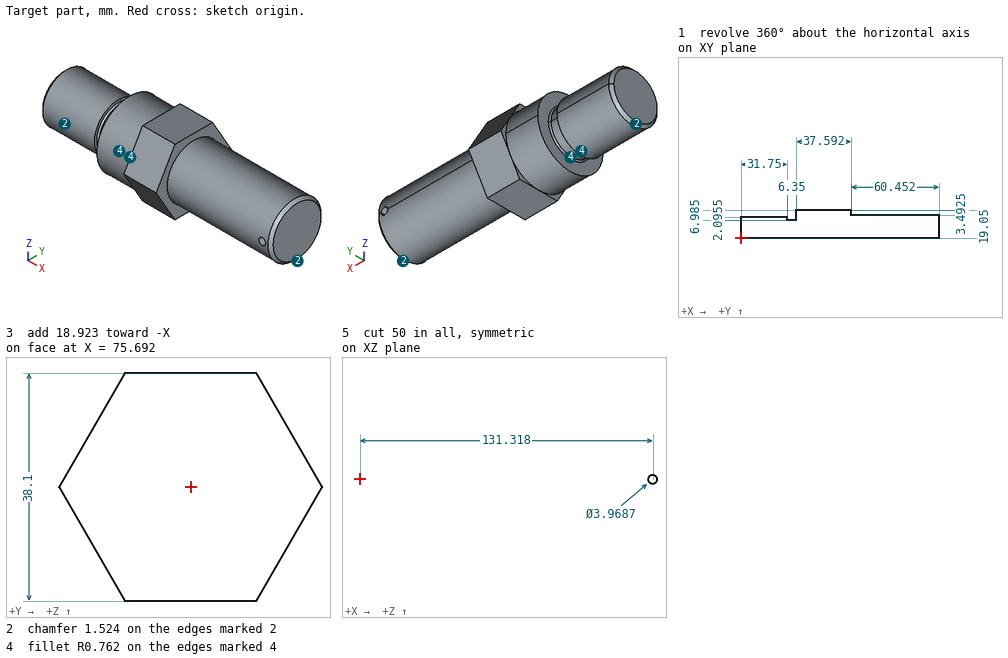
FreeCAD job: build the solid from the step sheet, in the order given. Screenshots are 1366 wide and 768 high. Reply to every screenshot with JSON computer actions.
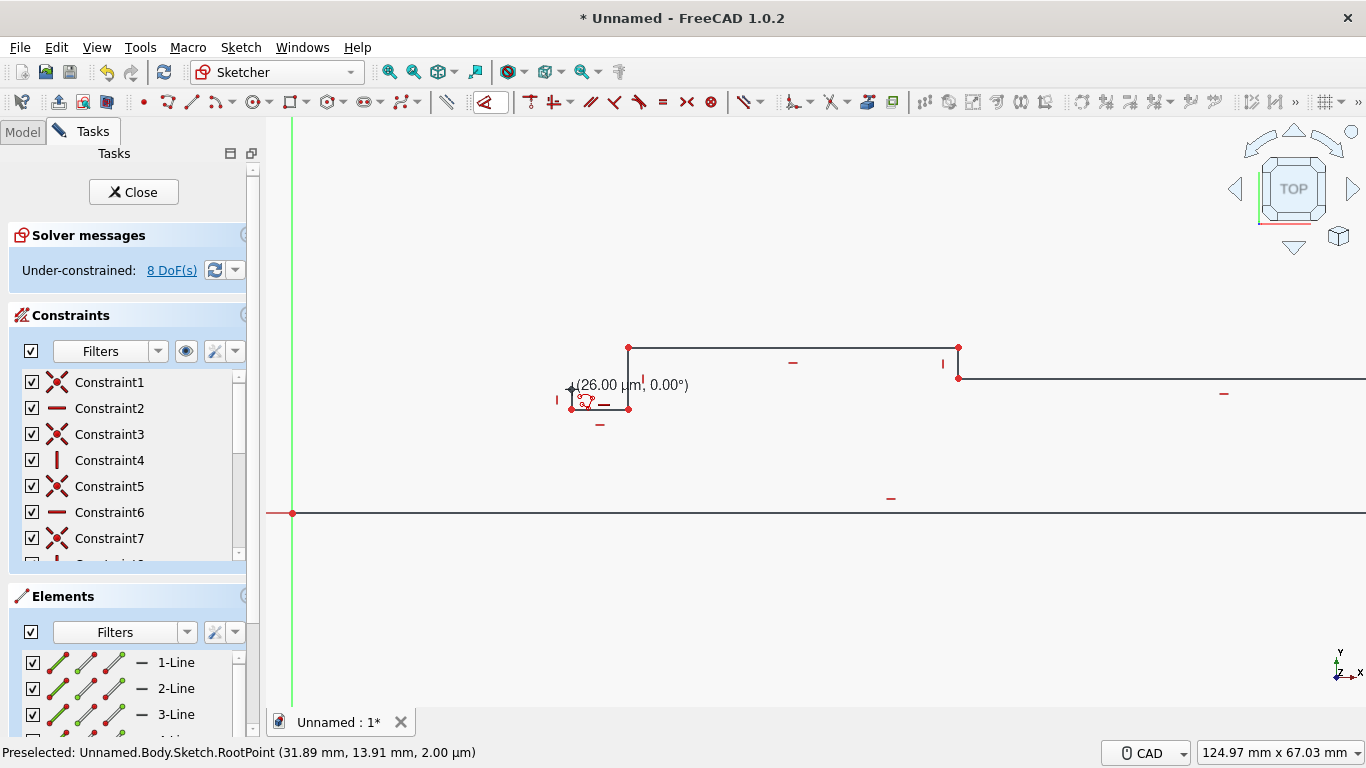
{"action": "scroll", "coordinate": [572, 391], "scroll_direction": "down", "scroll_amount": 3}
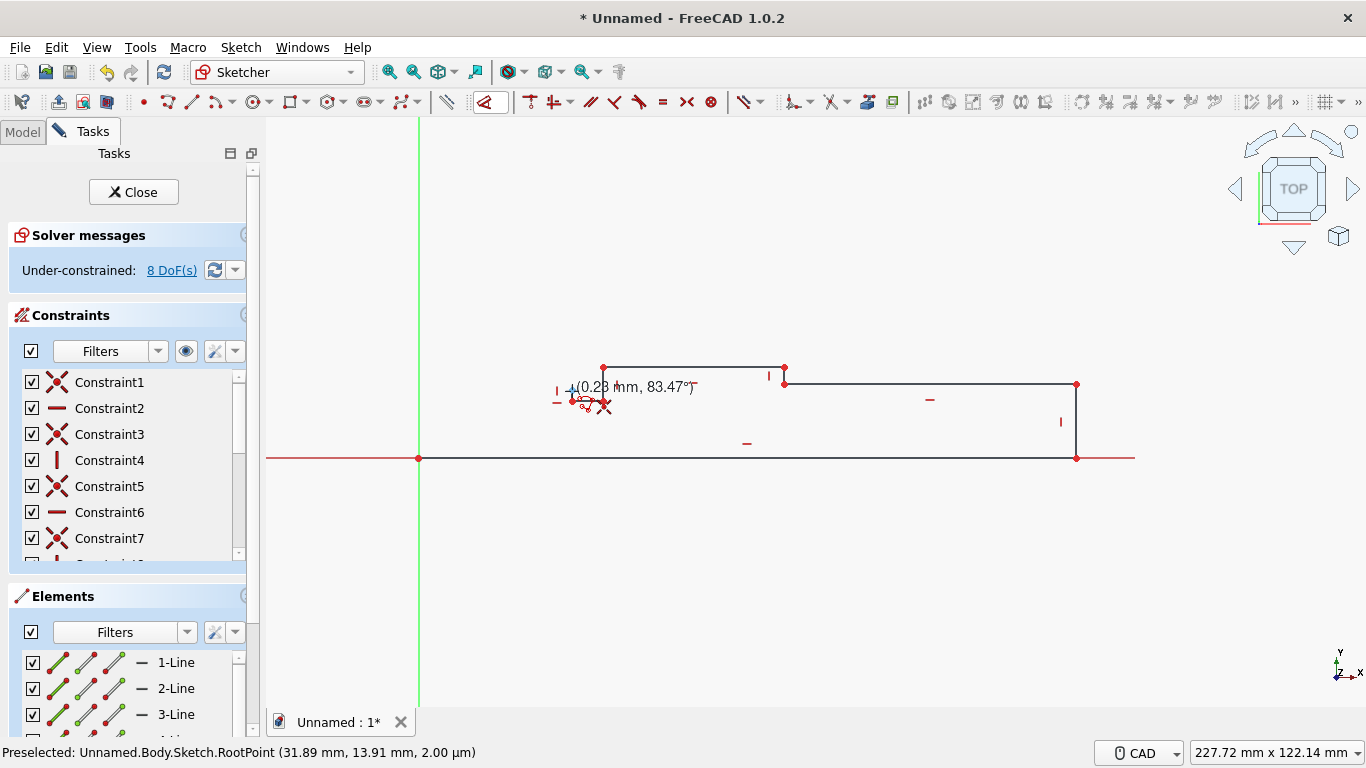
{"action": "left_click", "coordinate": [428, 390]}
{"action": "left_click", "coordinate": [419, 458]}
{"action": "key", "text": "Escape"}
{"action": "key", "text": "Escape"}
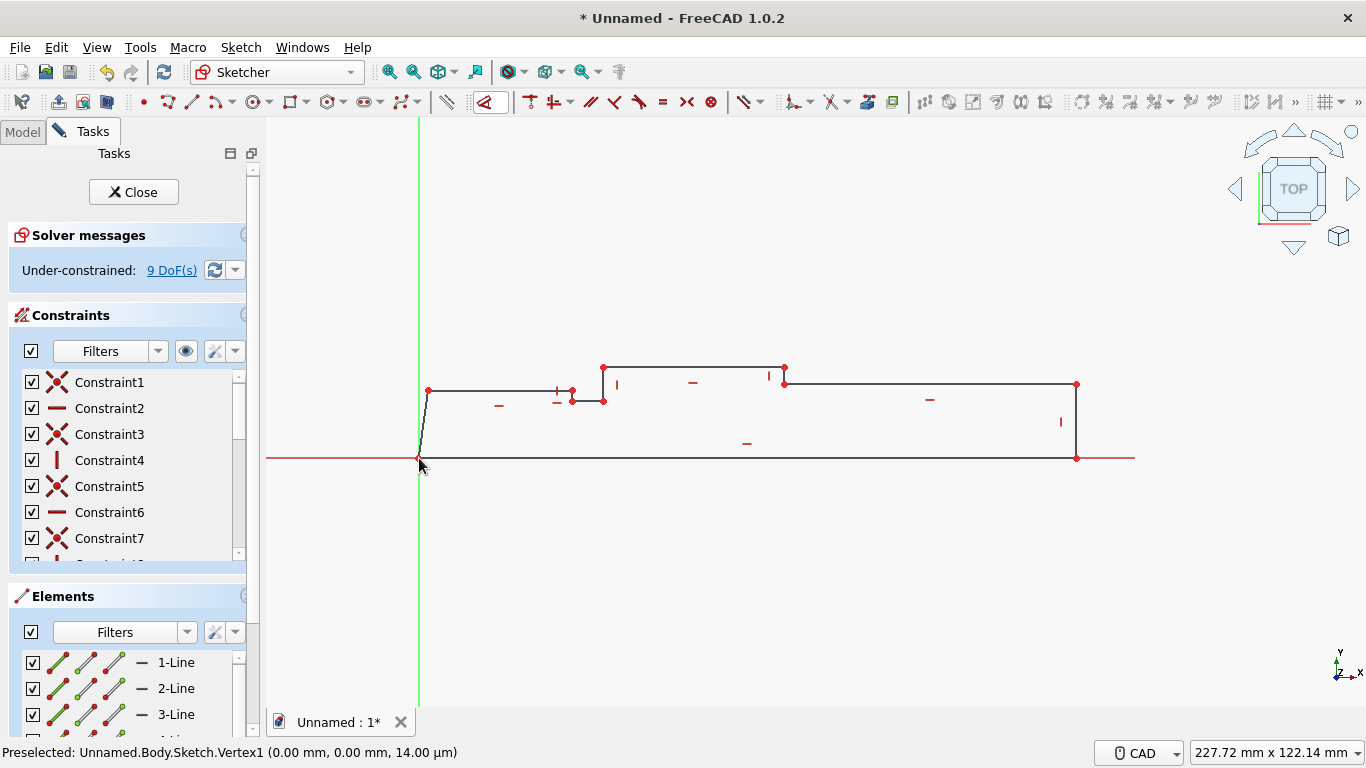
{"action": "left_click", "coordinate": [421, 438]}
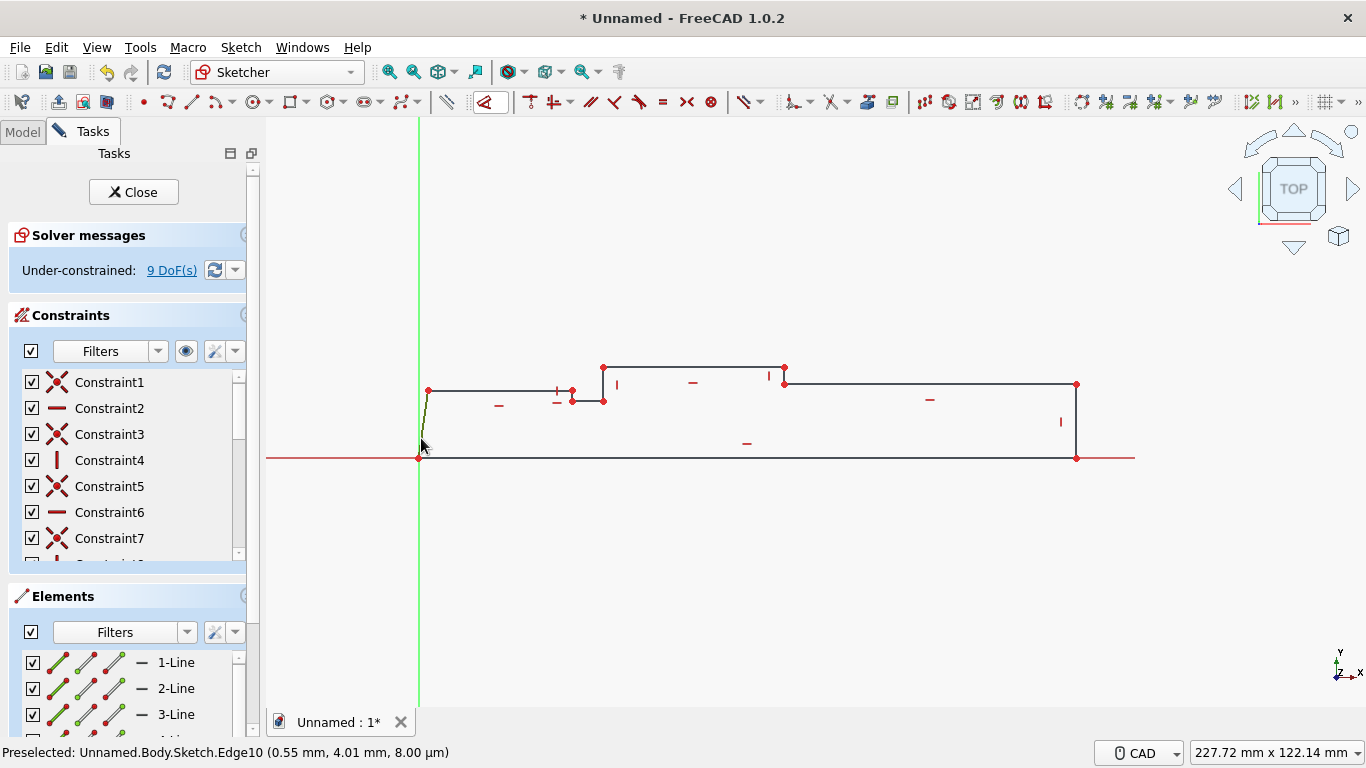
{"action": "key", "text": "v"}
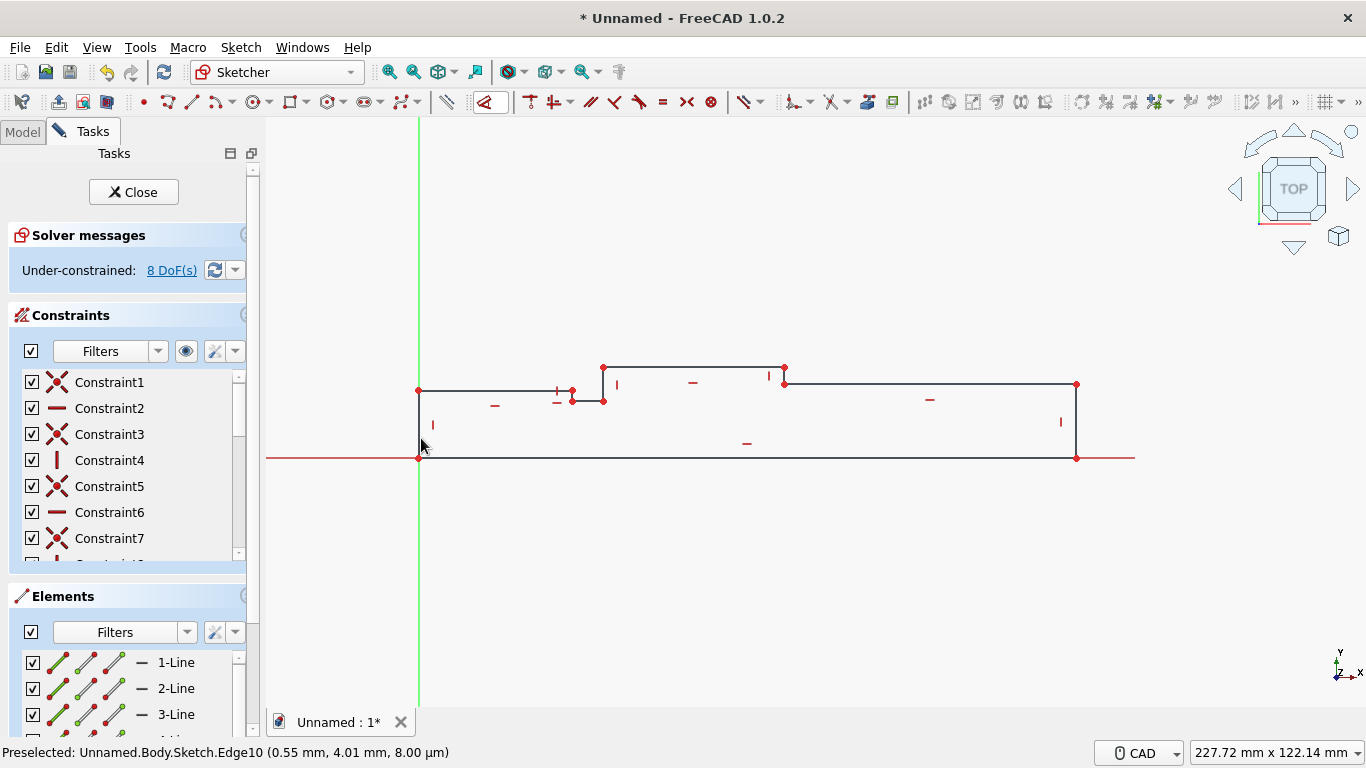
{"action": "key", "text": "d"}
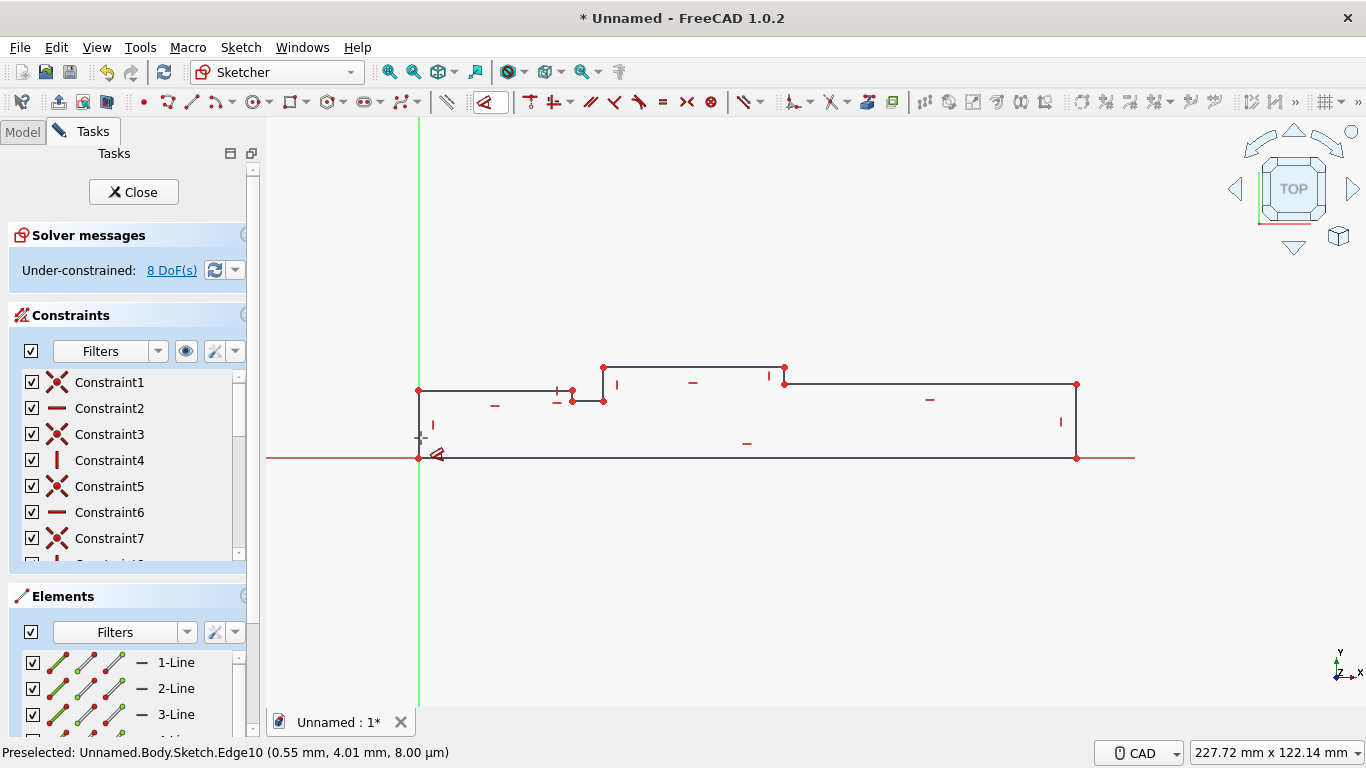
{"action": "scroll", "coordinate": [594, 401], "scroll_direction": "up", "scroll_amount": 2}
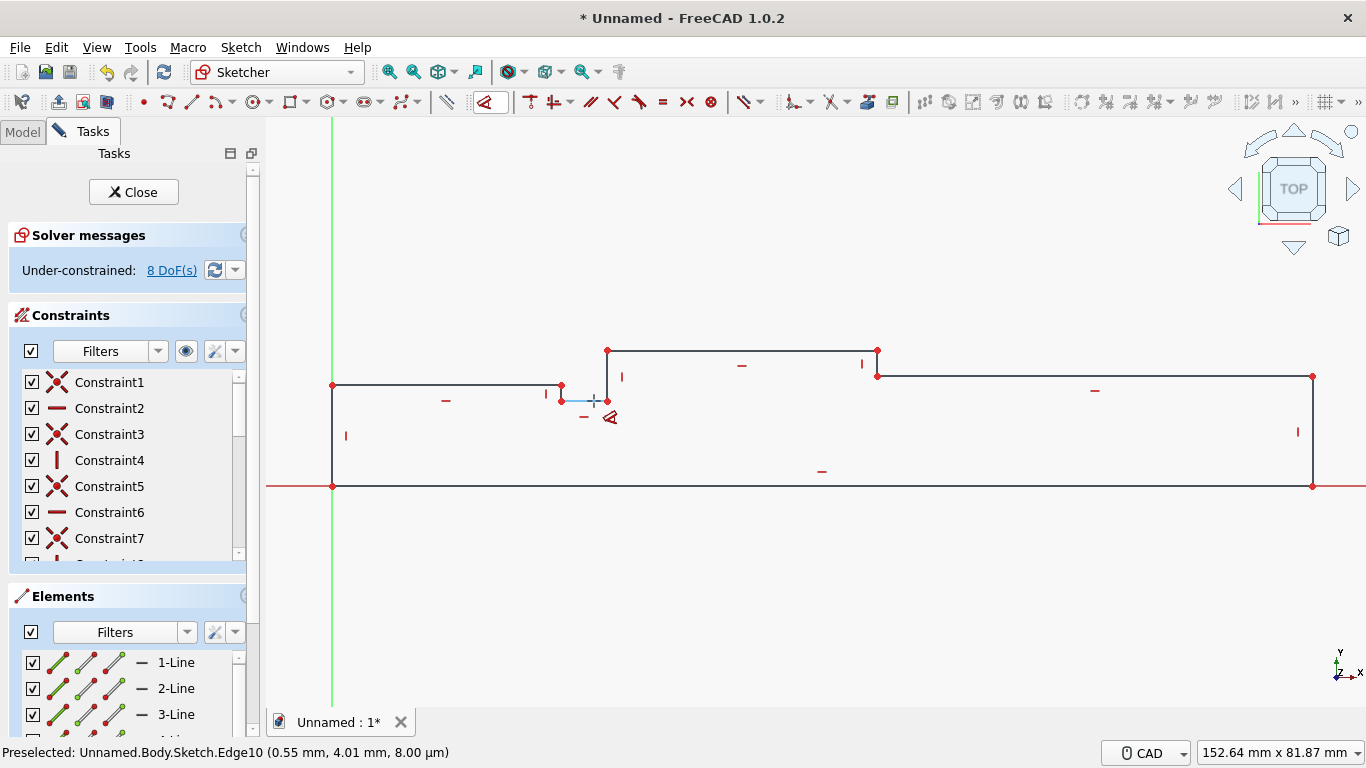
{"action": "left_click", "coordinate": [593, 401]}
{"action": "left_click", "coordinate": [584, 367]}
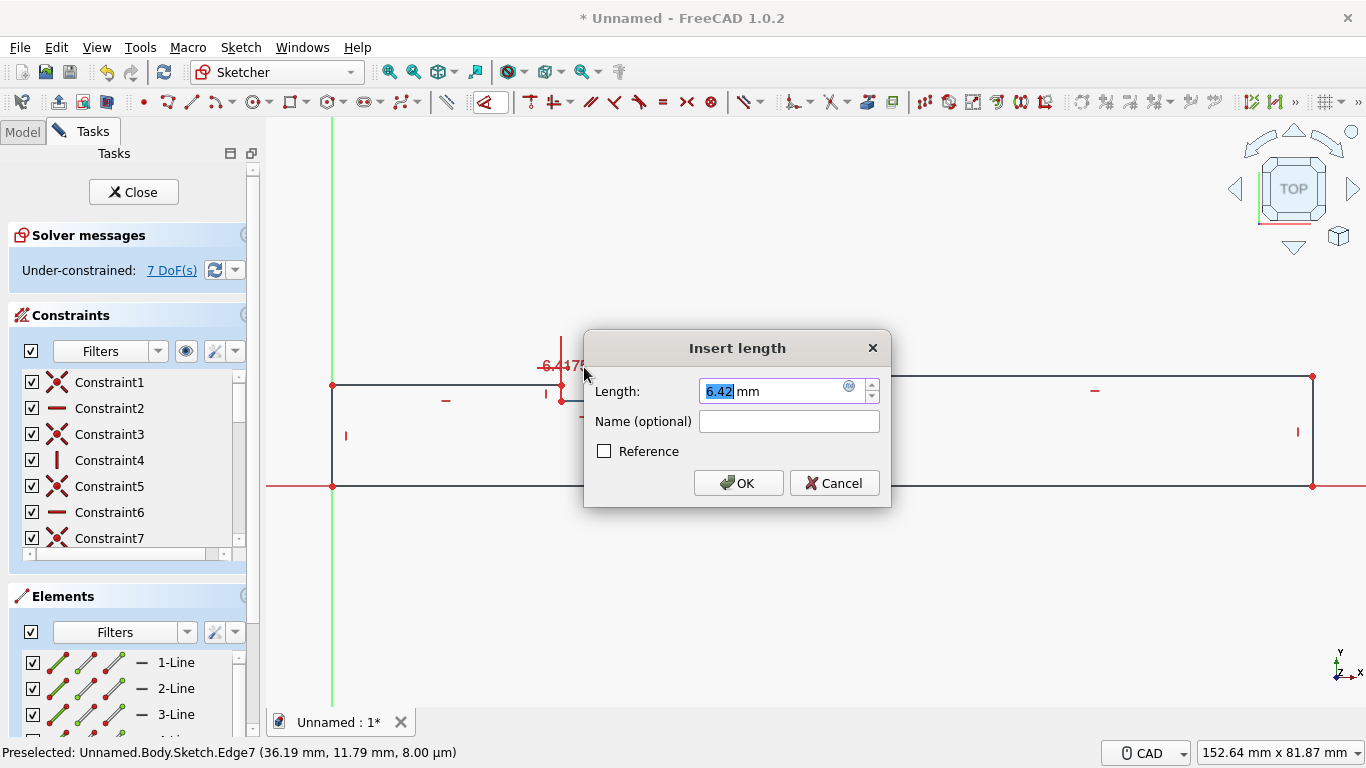
{"action": "type", "text": "6.35"}
{"action": "key", "text": "Return"}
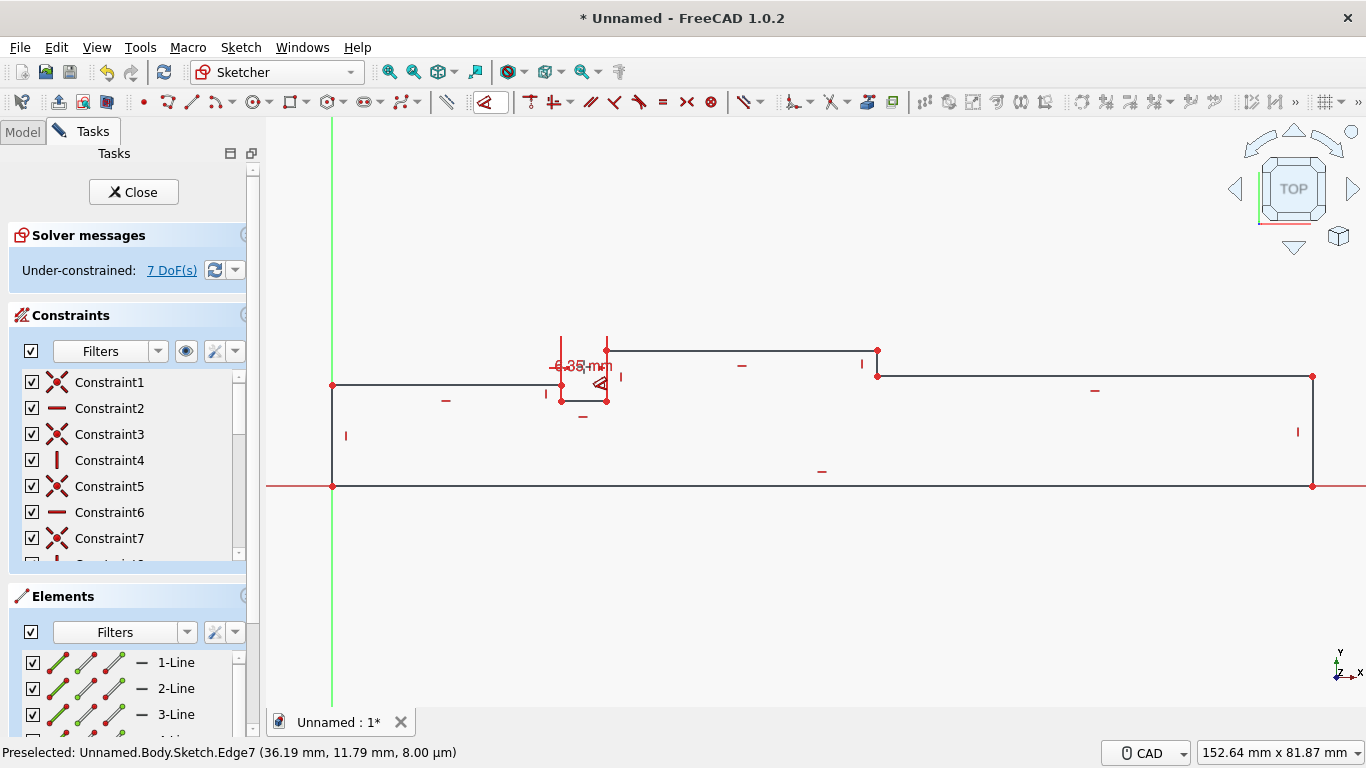
{"action": "left_click", "coordinate": [607, 366]}
{"action": "left_click", "coordinate": [641, 388]}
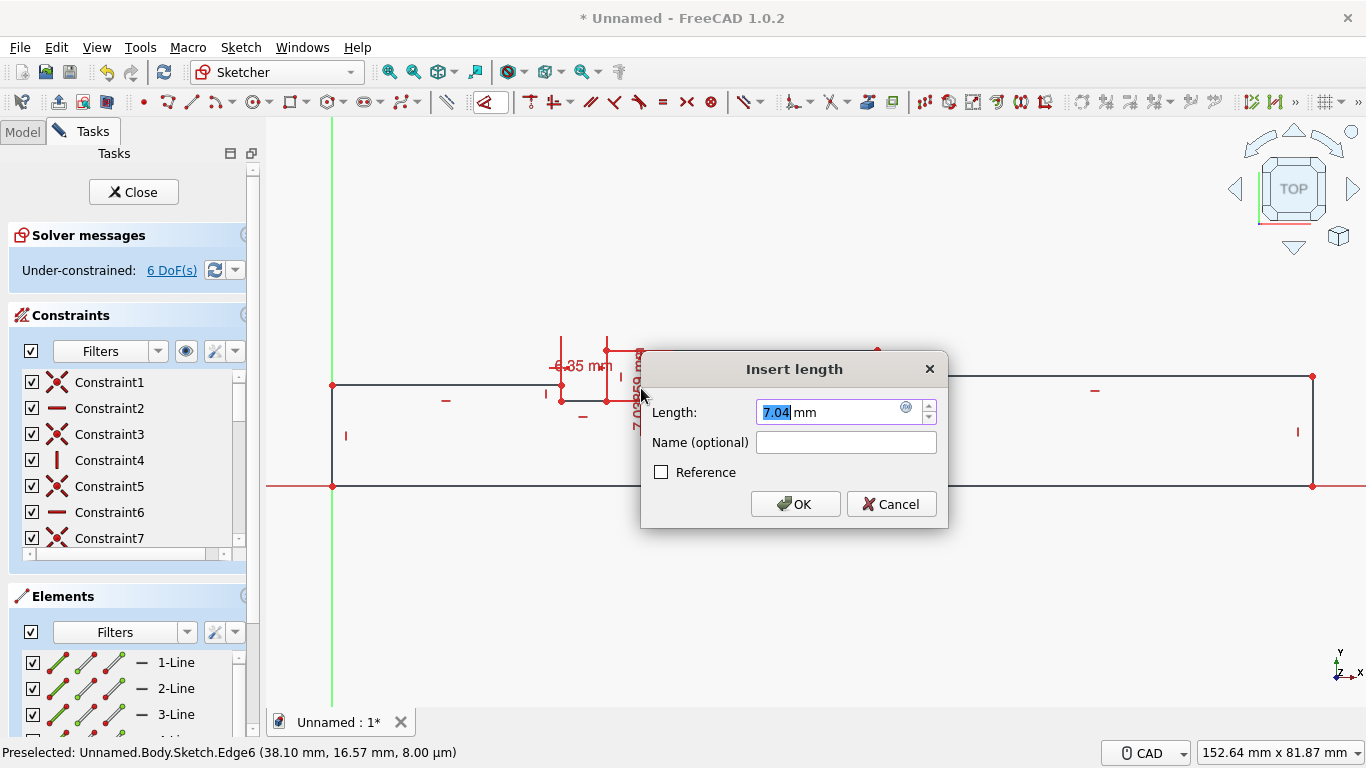
{"action": "type", "text": "6.985"}
{"action": "key", "text": "Return"}